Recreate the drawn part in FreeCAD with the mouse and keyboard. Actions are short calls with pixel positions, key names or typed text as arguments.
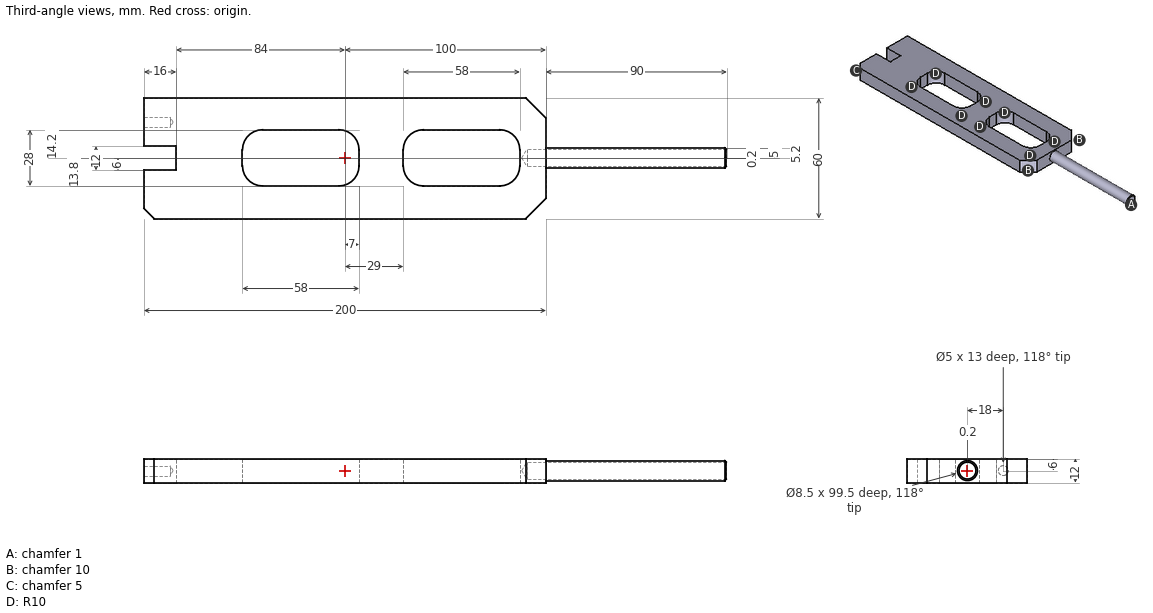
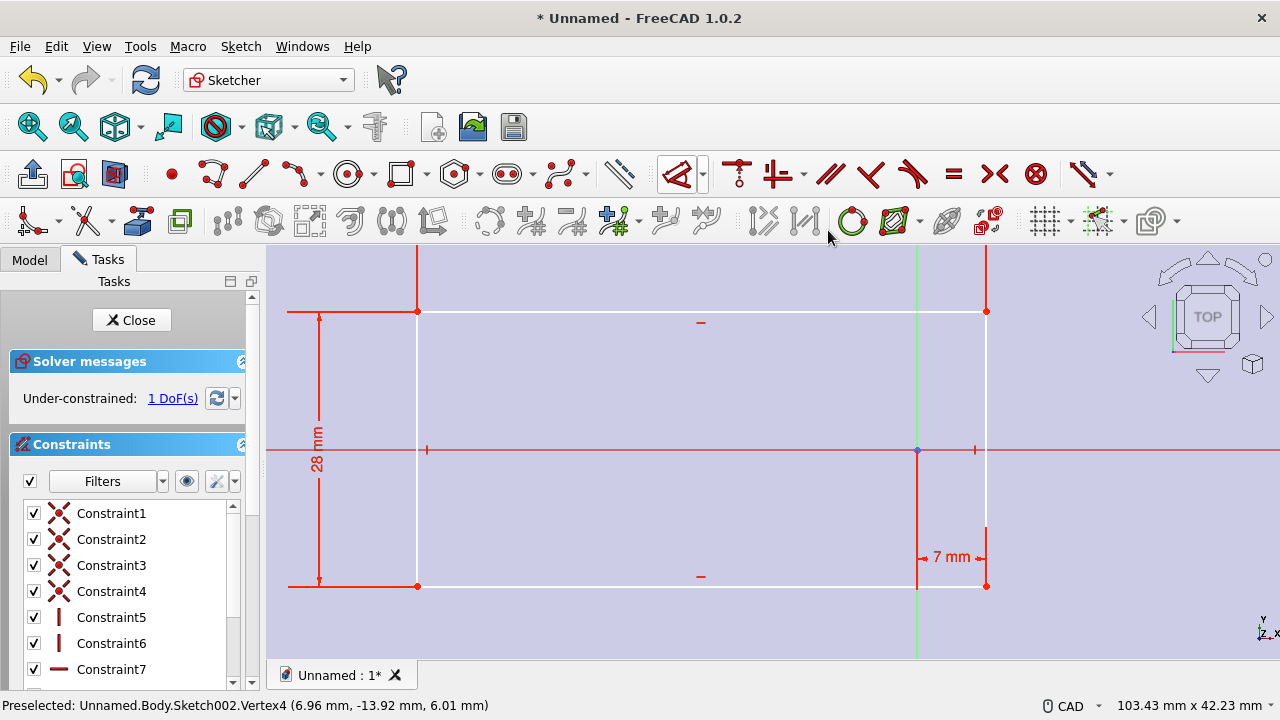
click(417, 312)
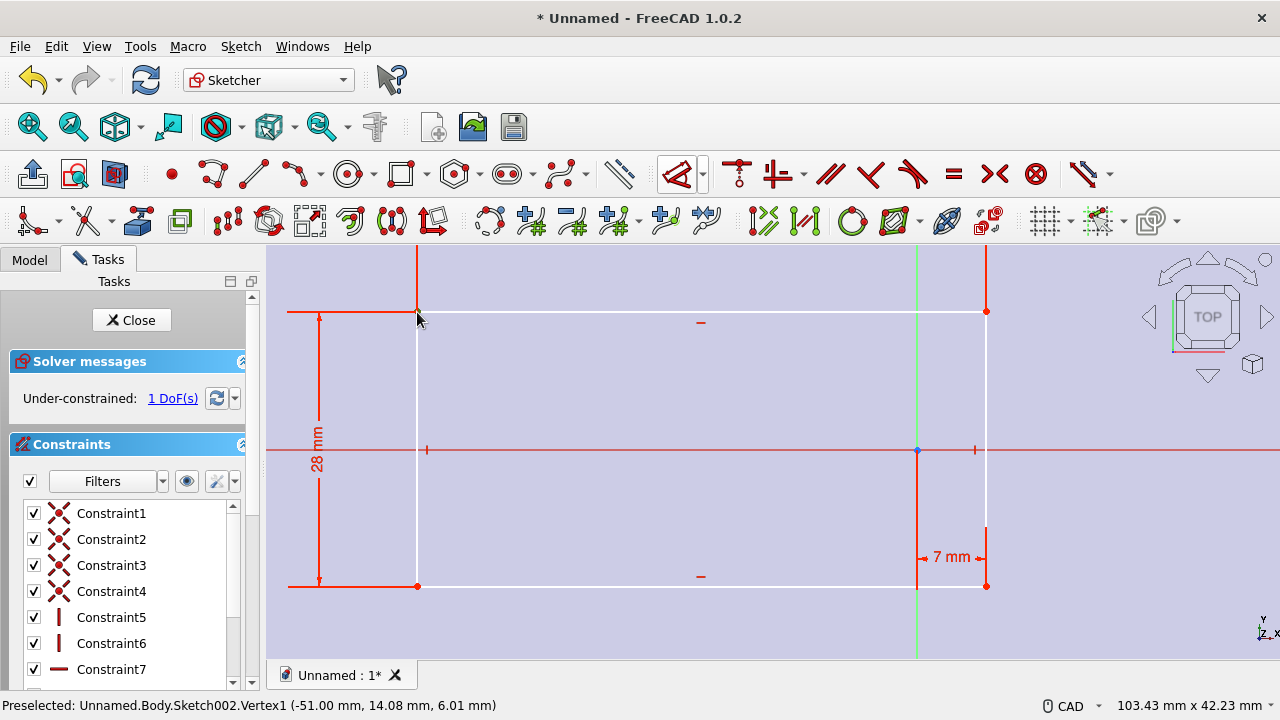
key(i)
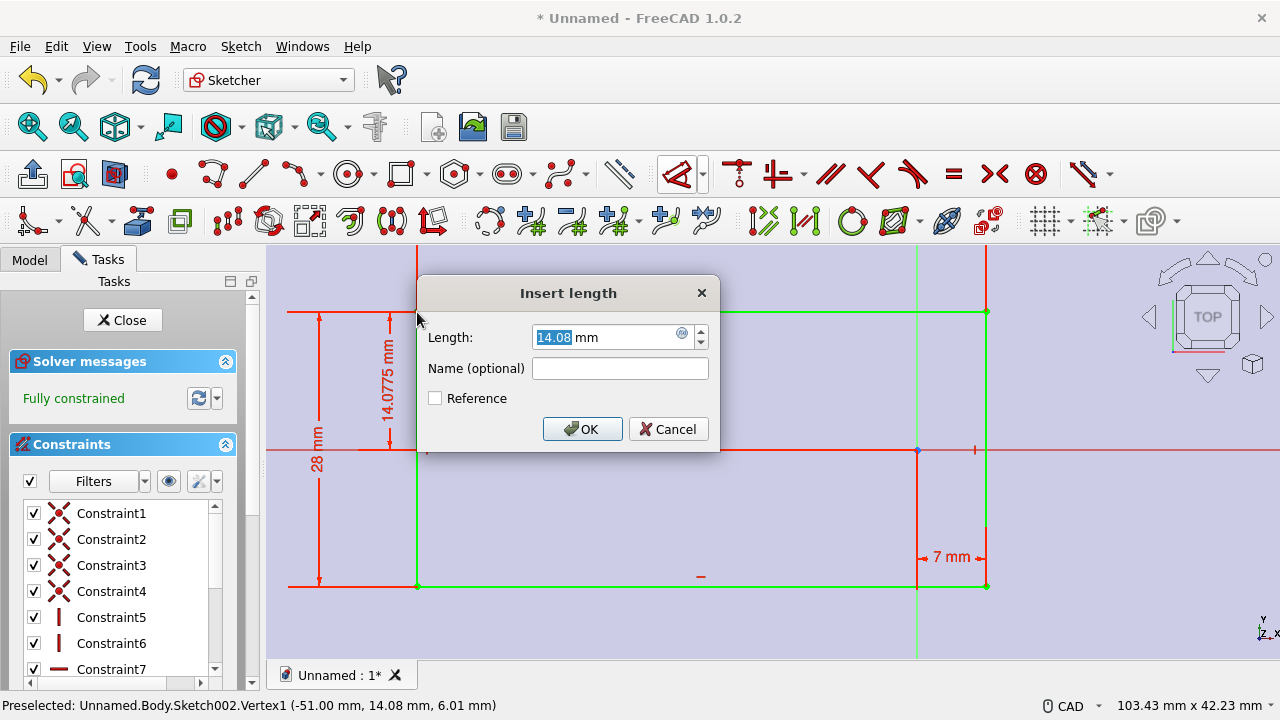
text(14.2)
key(Return)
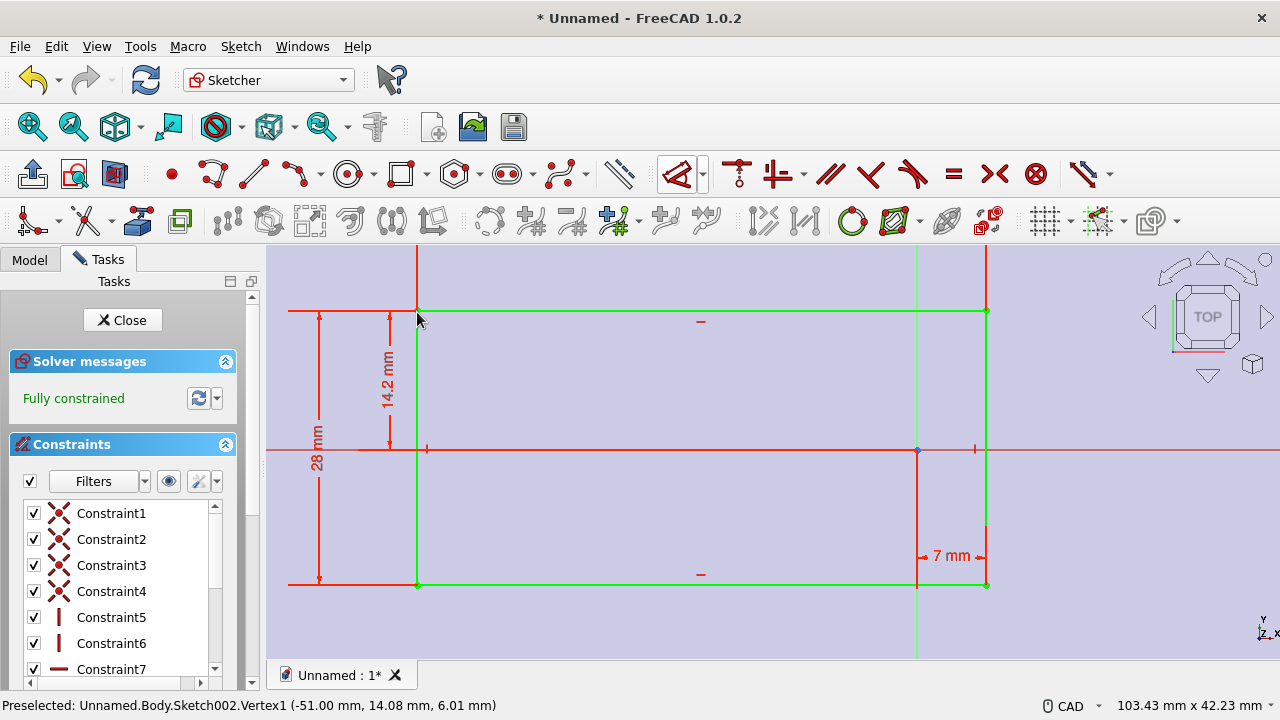
click(123, 320)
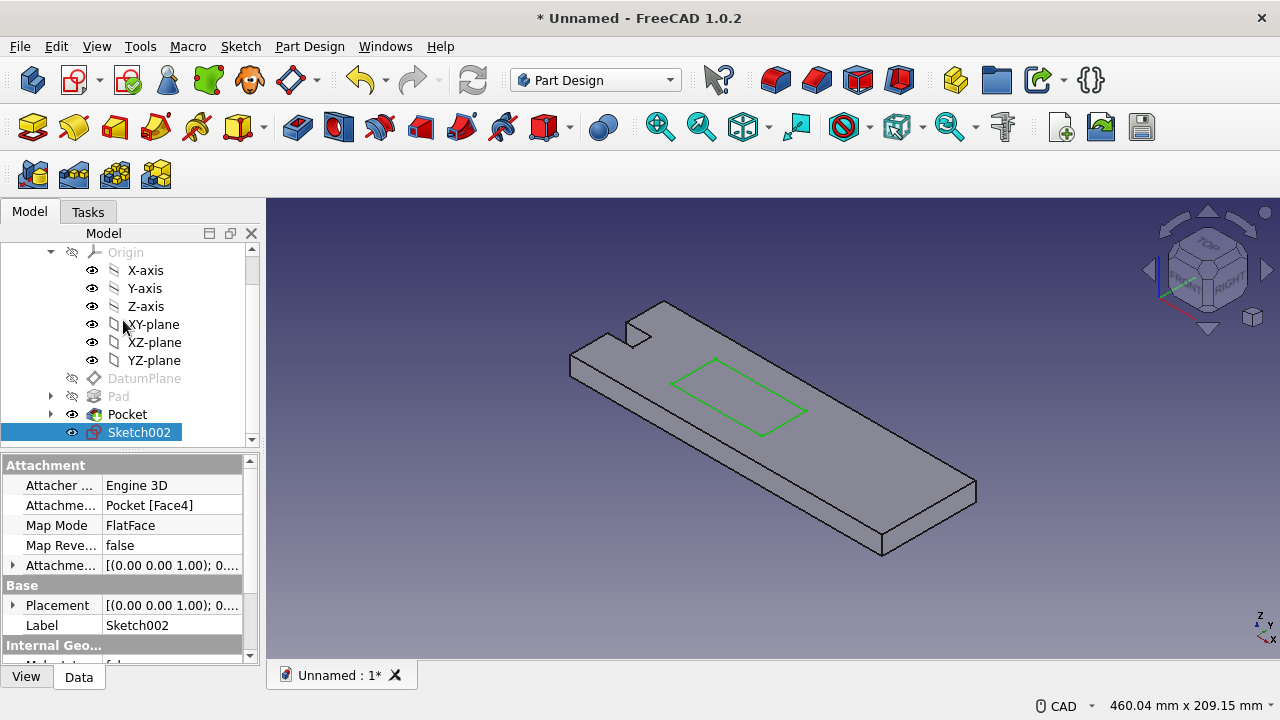
click(298, 128)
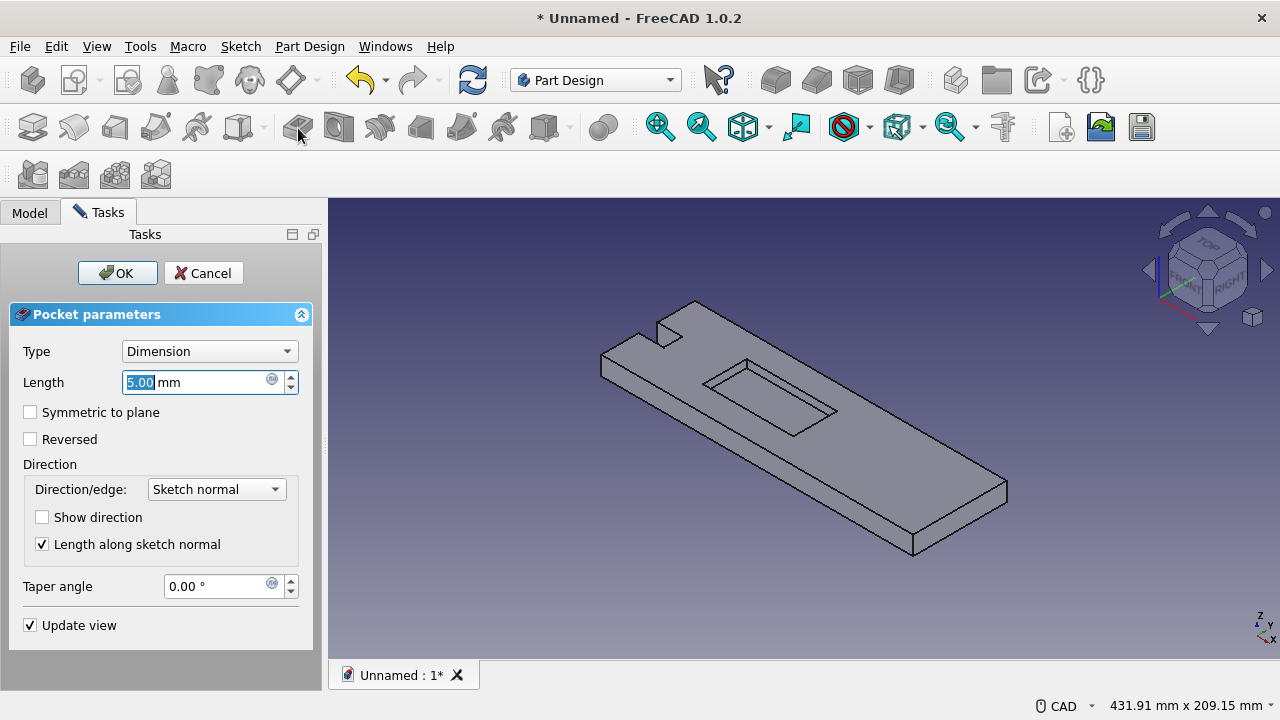
click(210, 352)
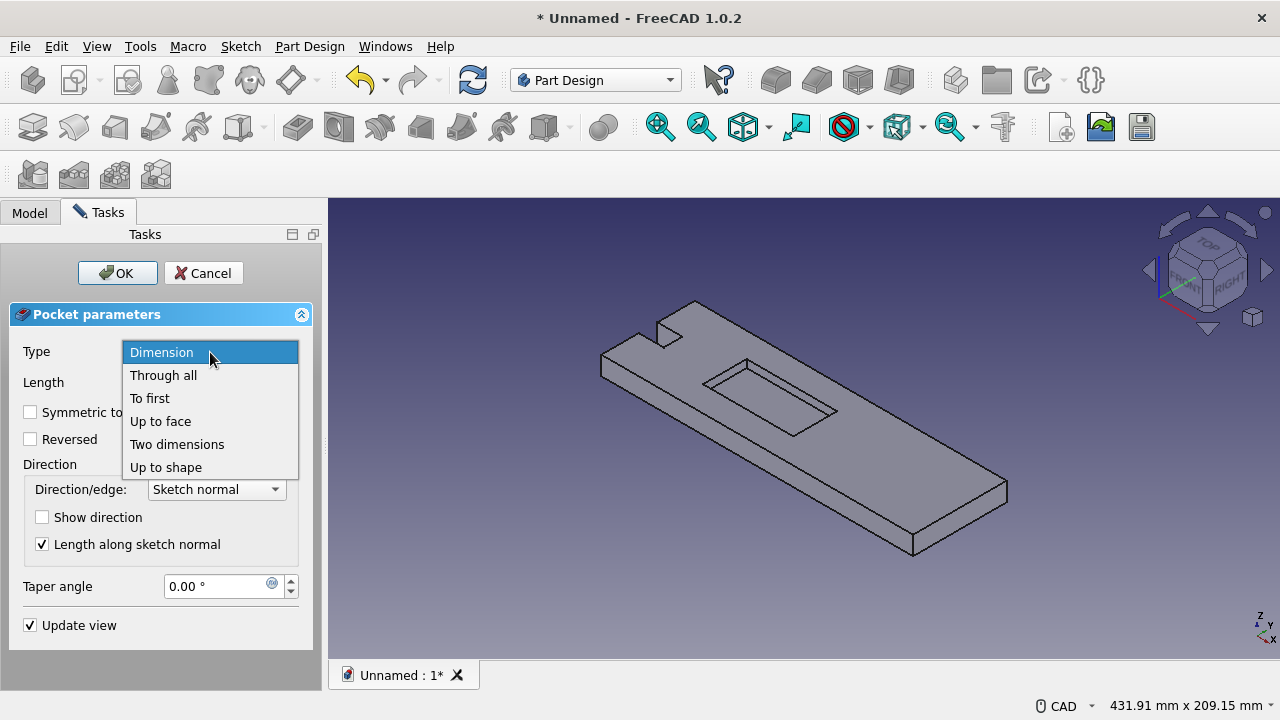
click(208, 376)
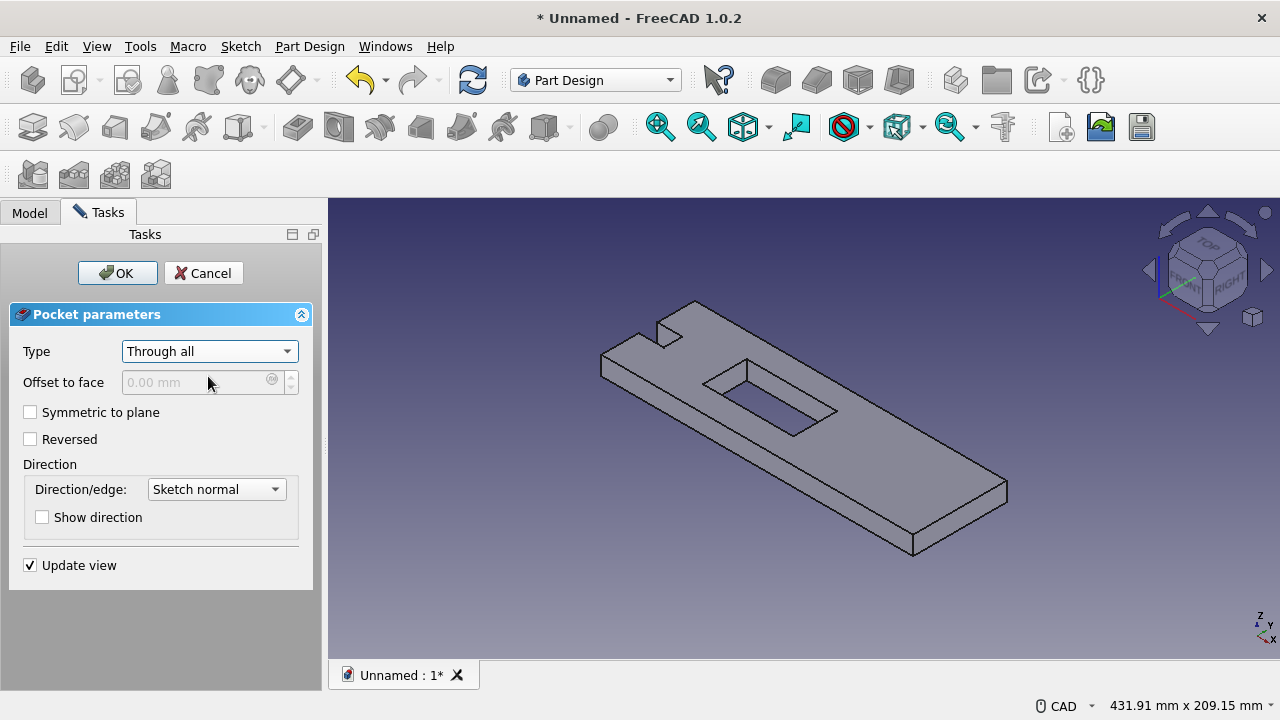
click(118, 273)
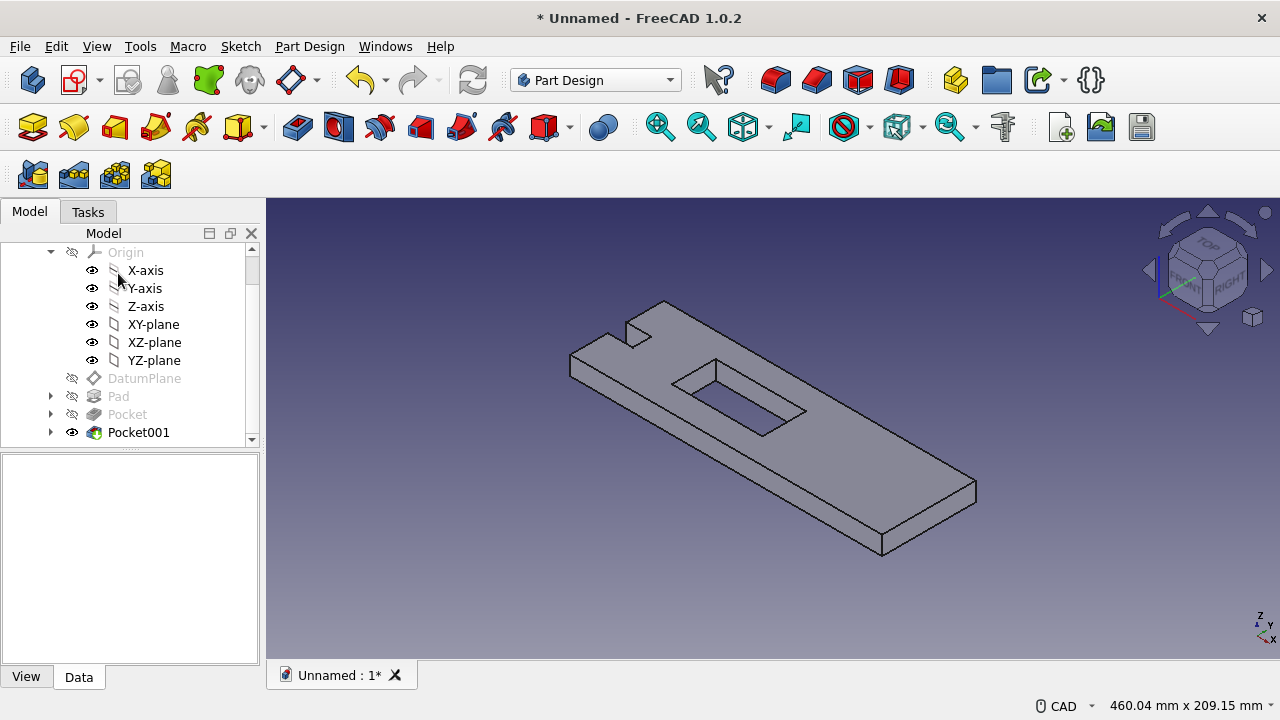
key(5)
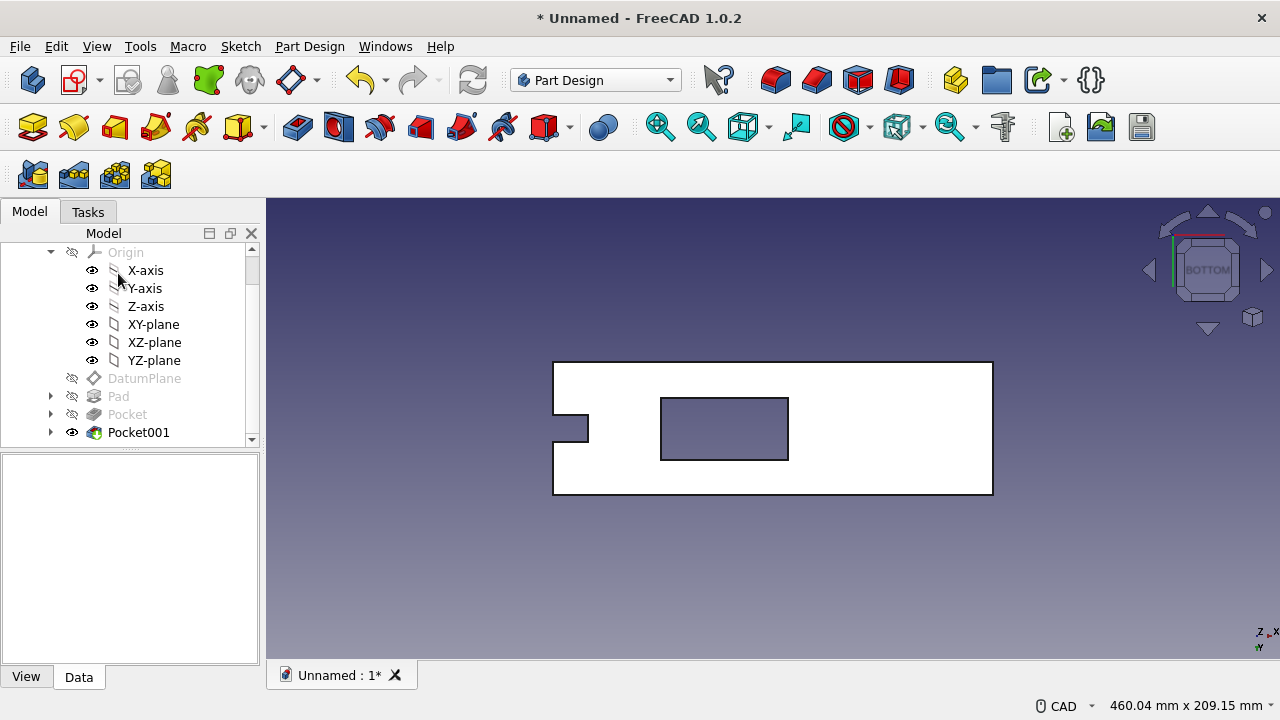
key(v)
key(f)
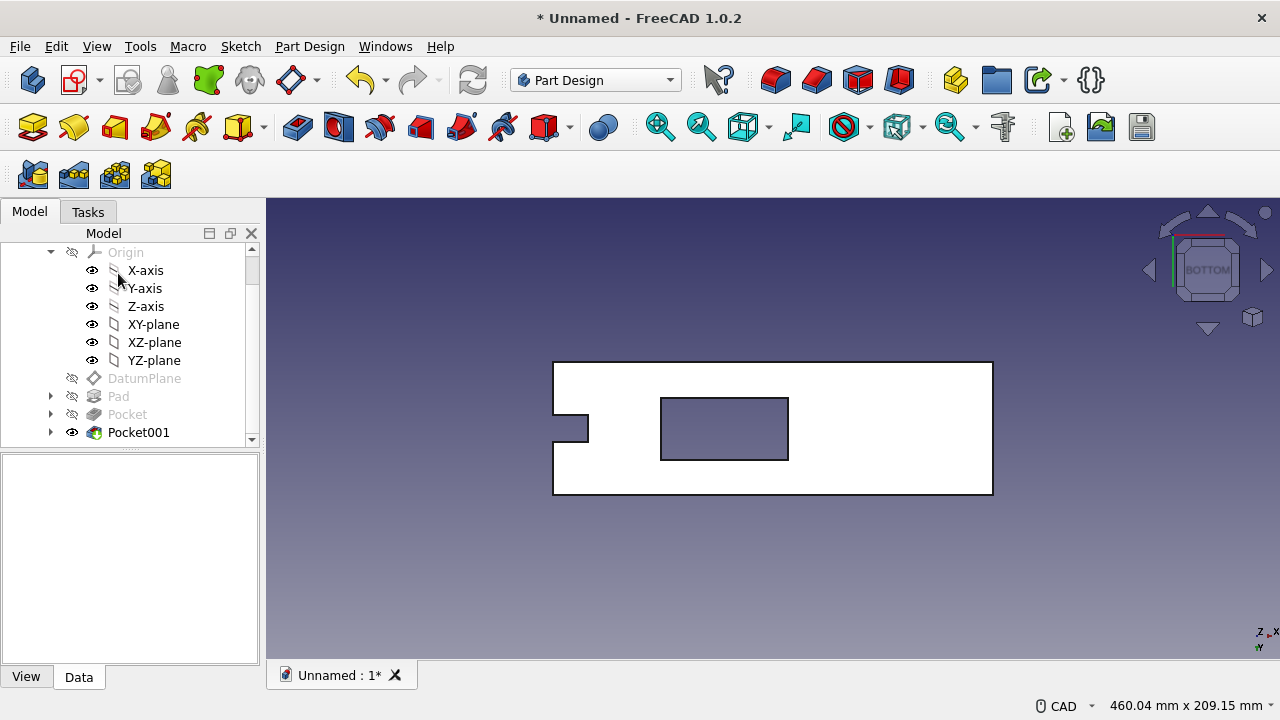
click(899, 427)